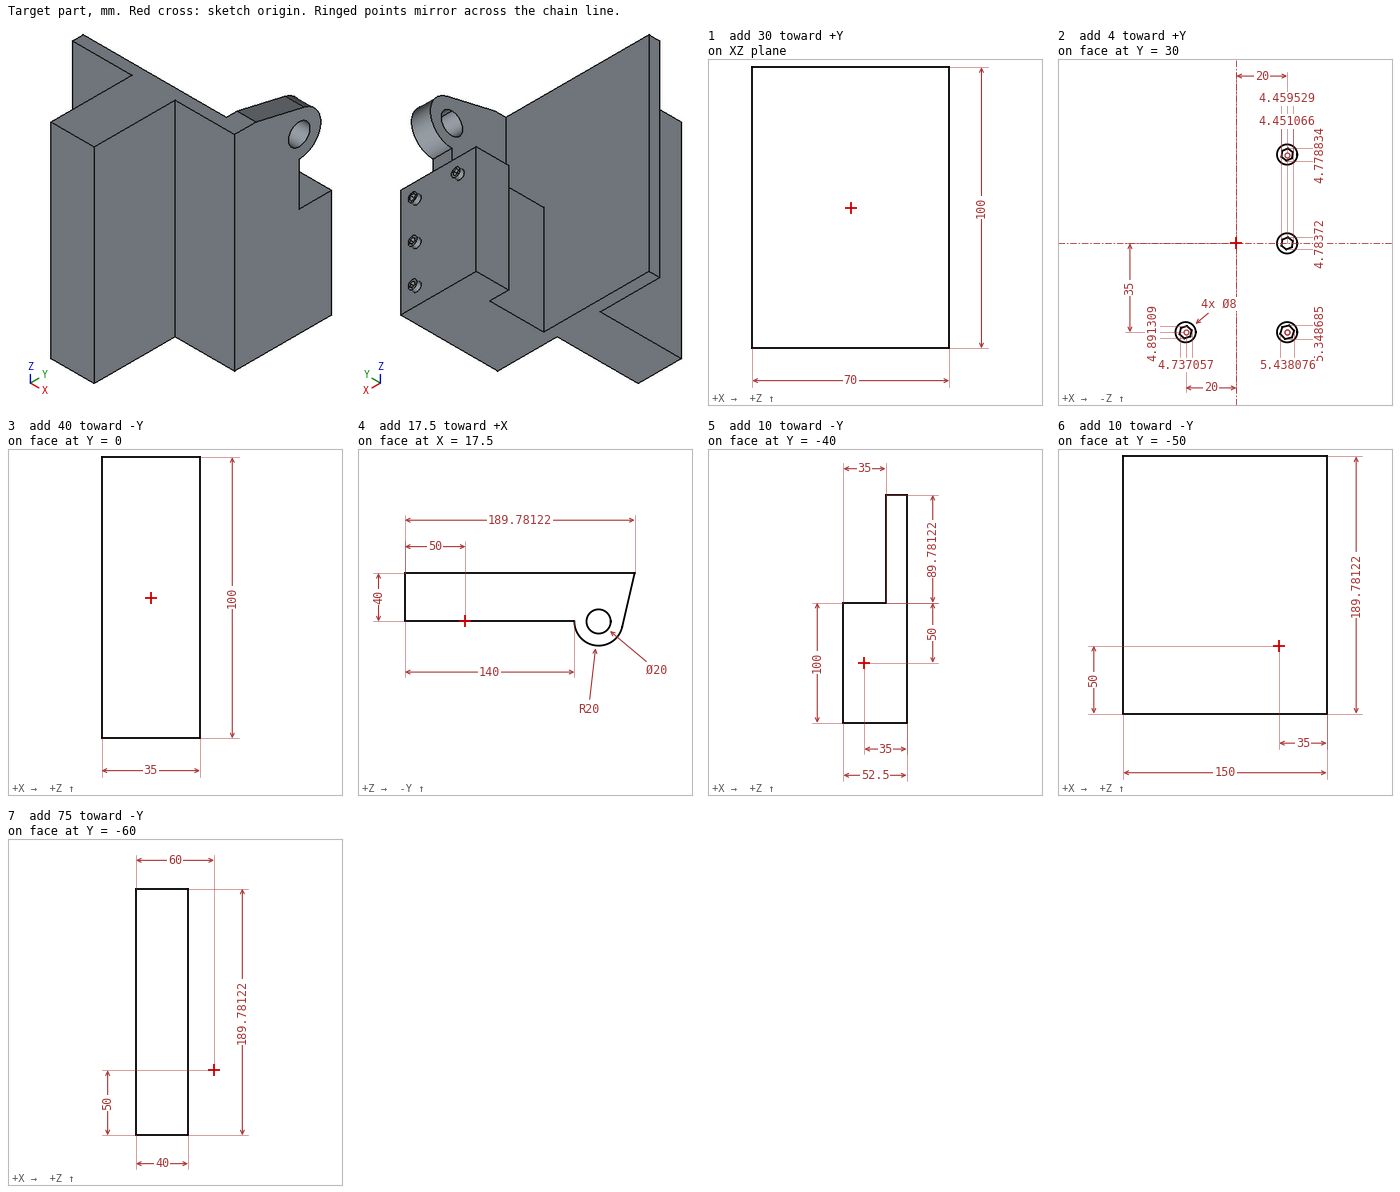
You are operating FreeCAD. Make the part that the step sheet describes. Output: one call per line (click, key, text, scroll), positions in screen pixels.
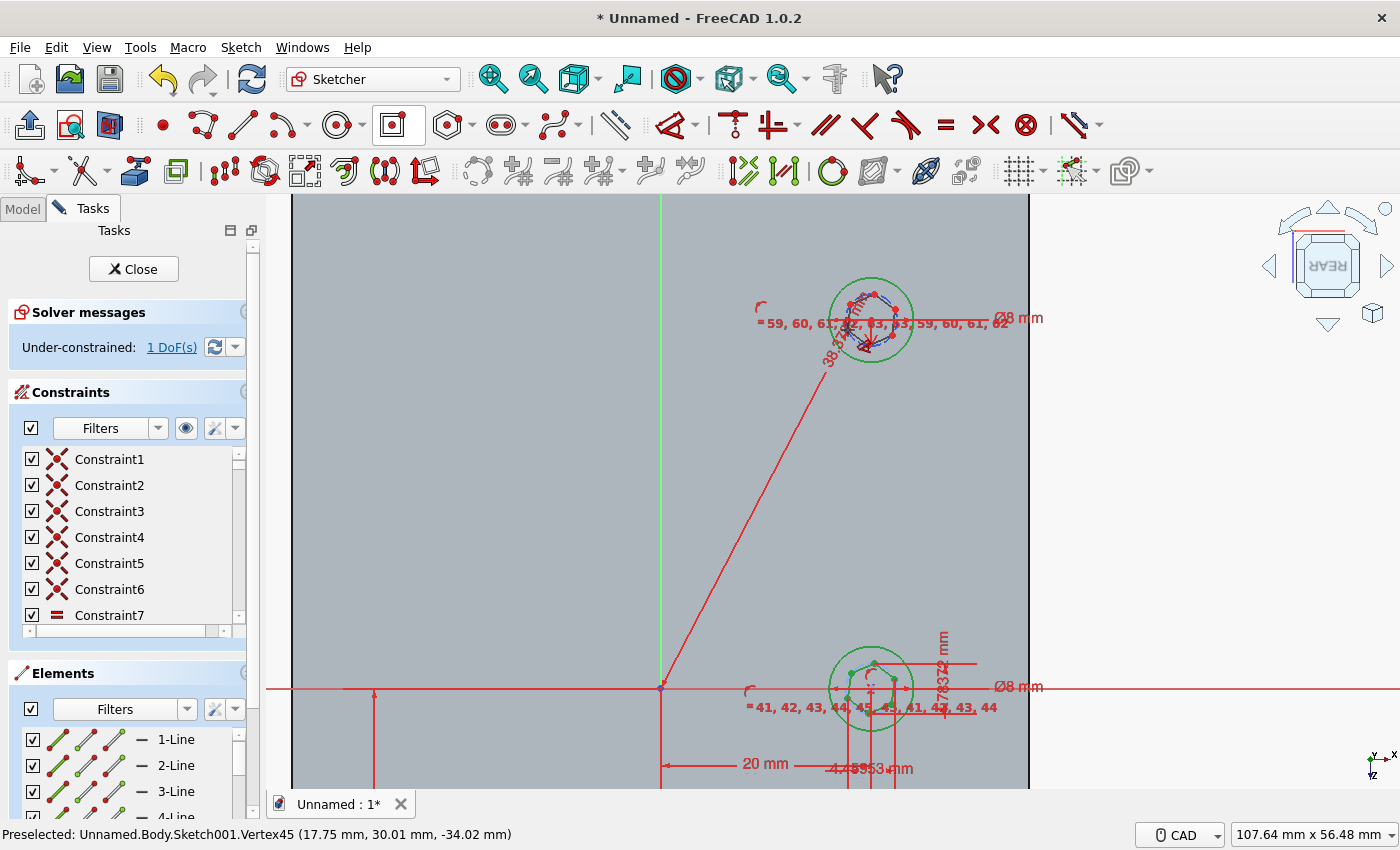
click(895, 310)
click(871, 252)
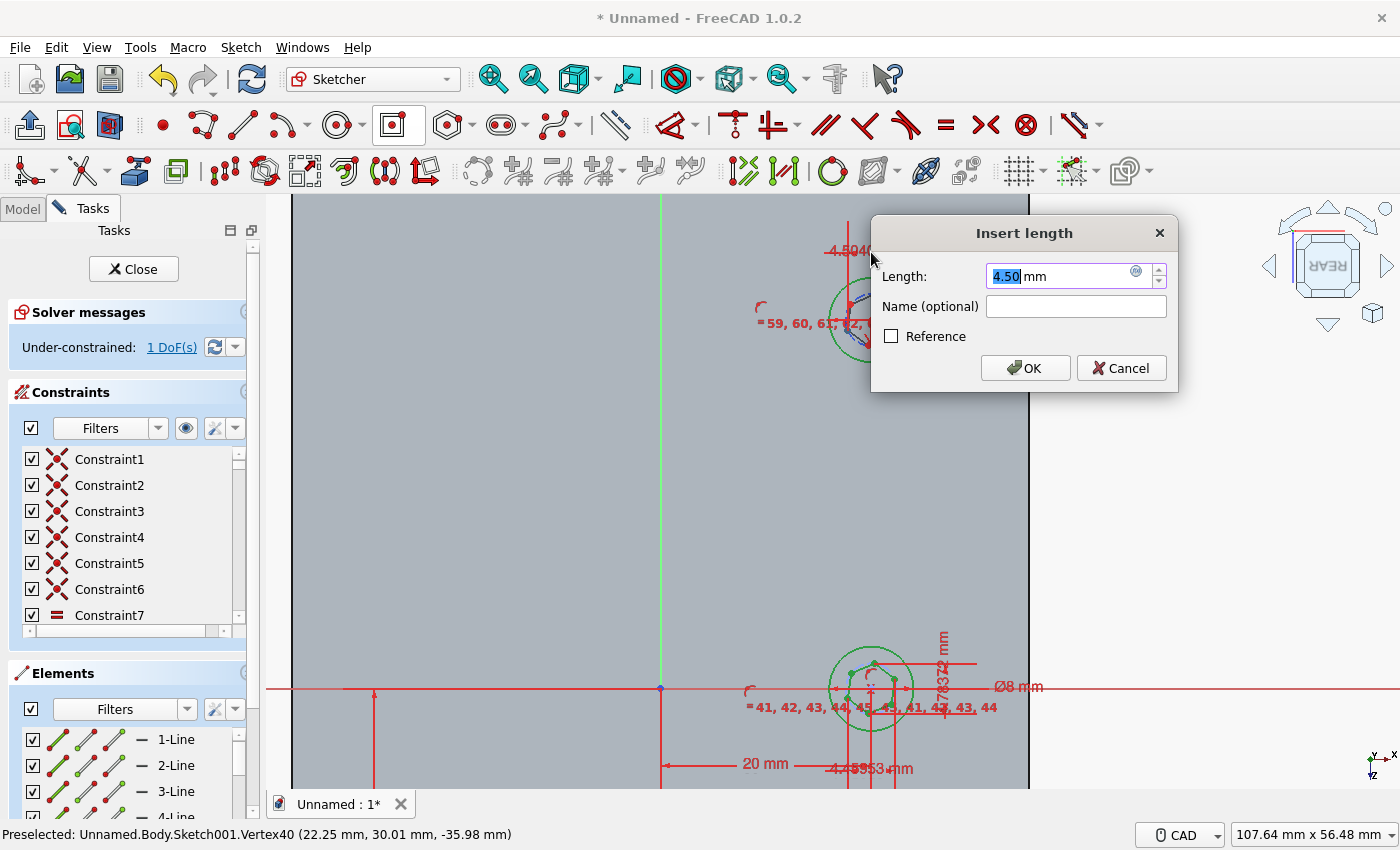
text(4.451066)
key(Return)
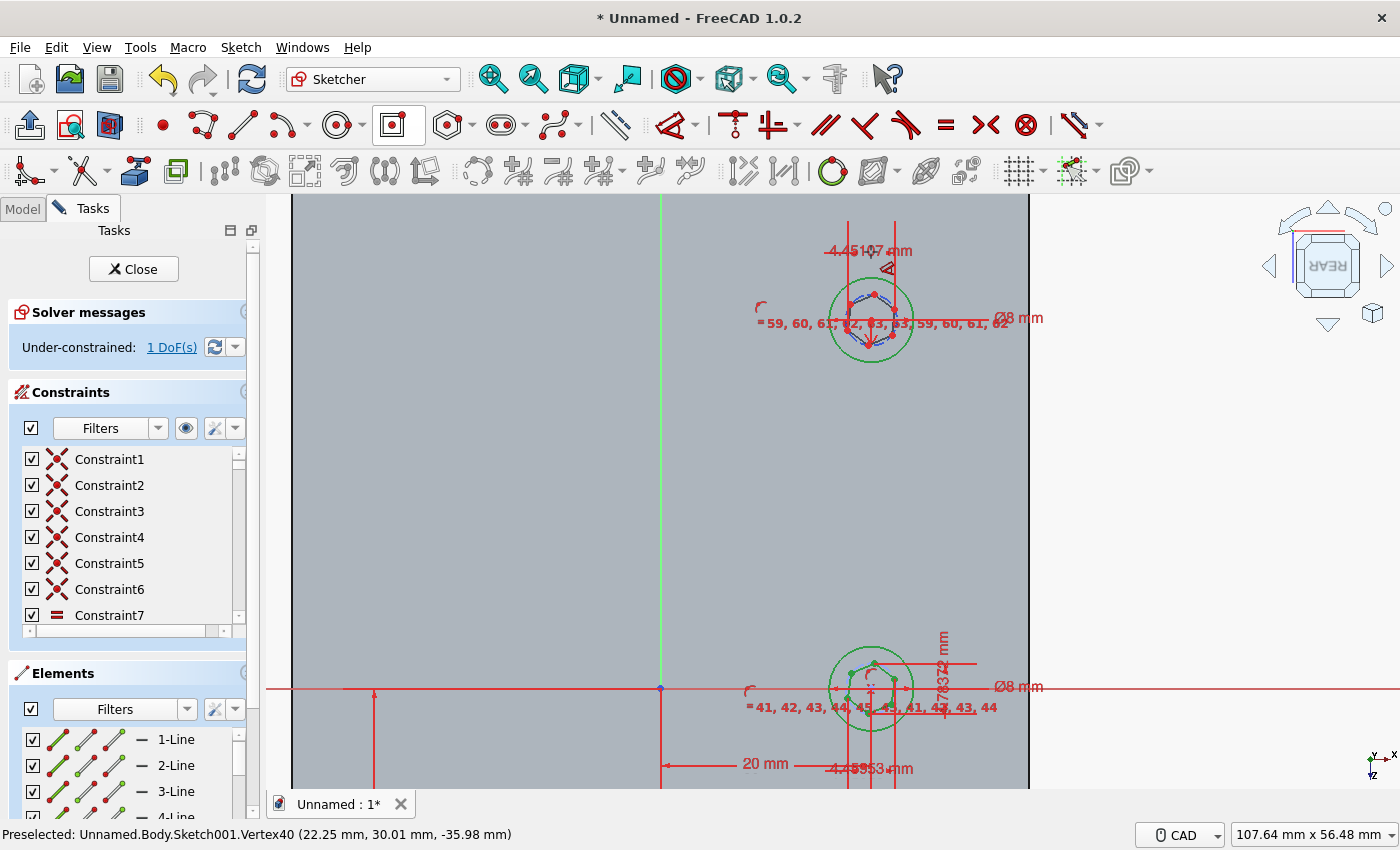
click(869, 346)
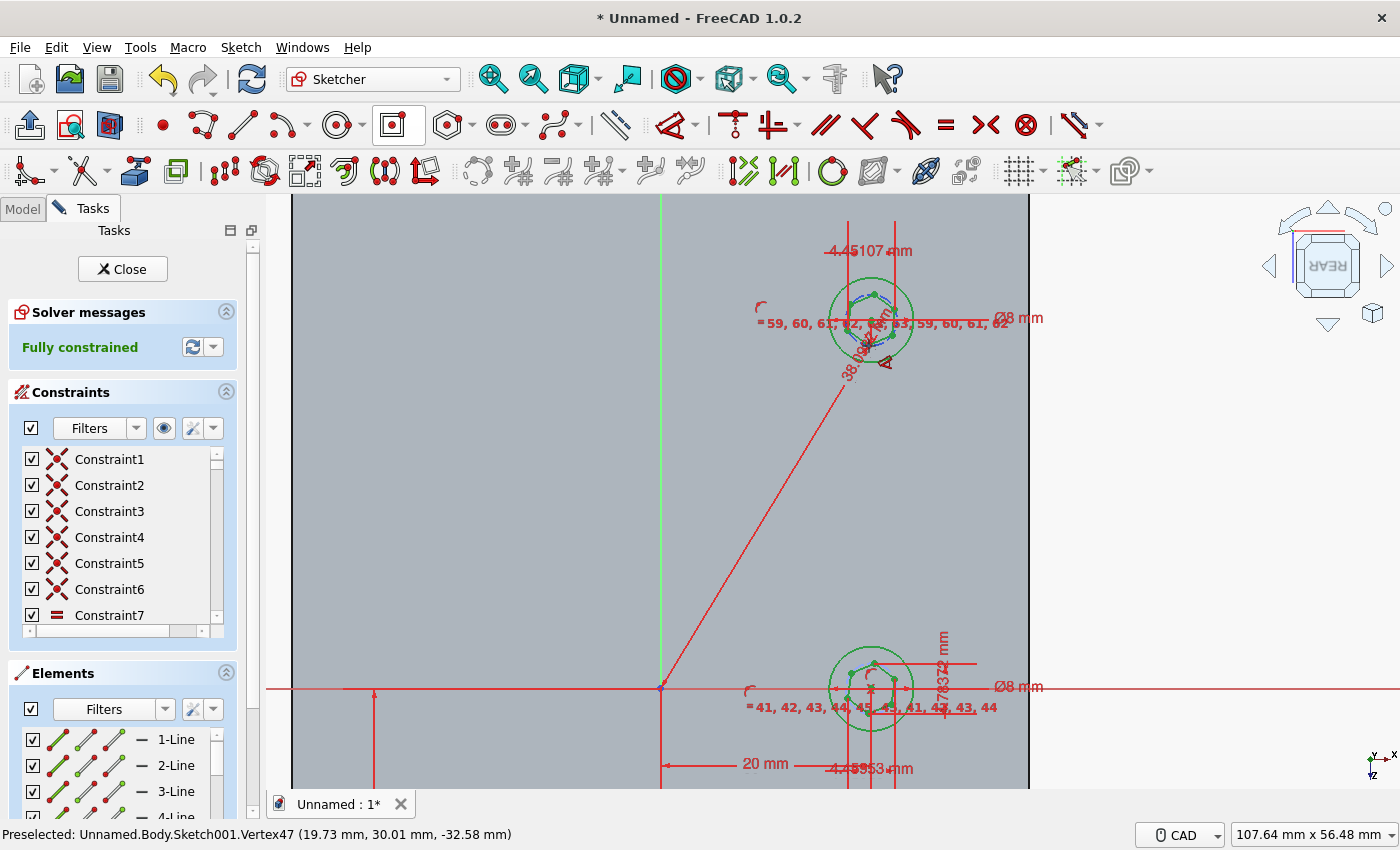
click(874, 295)
click(932, 320)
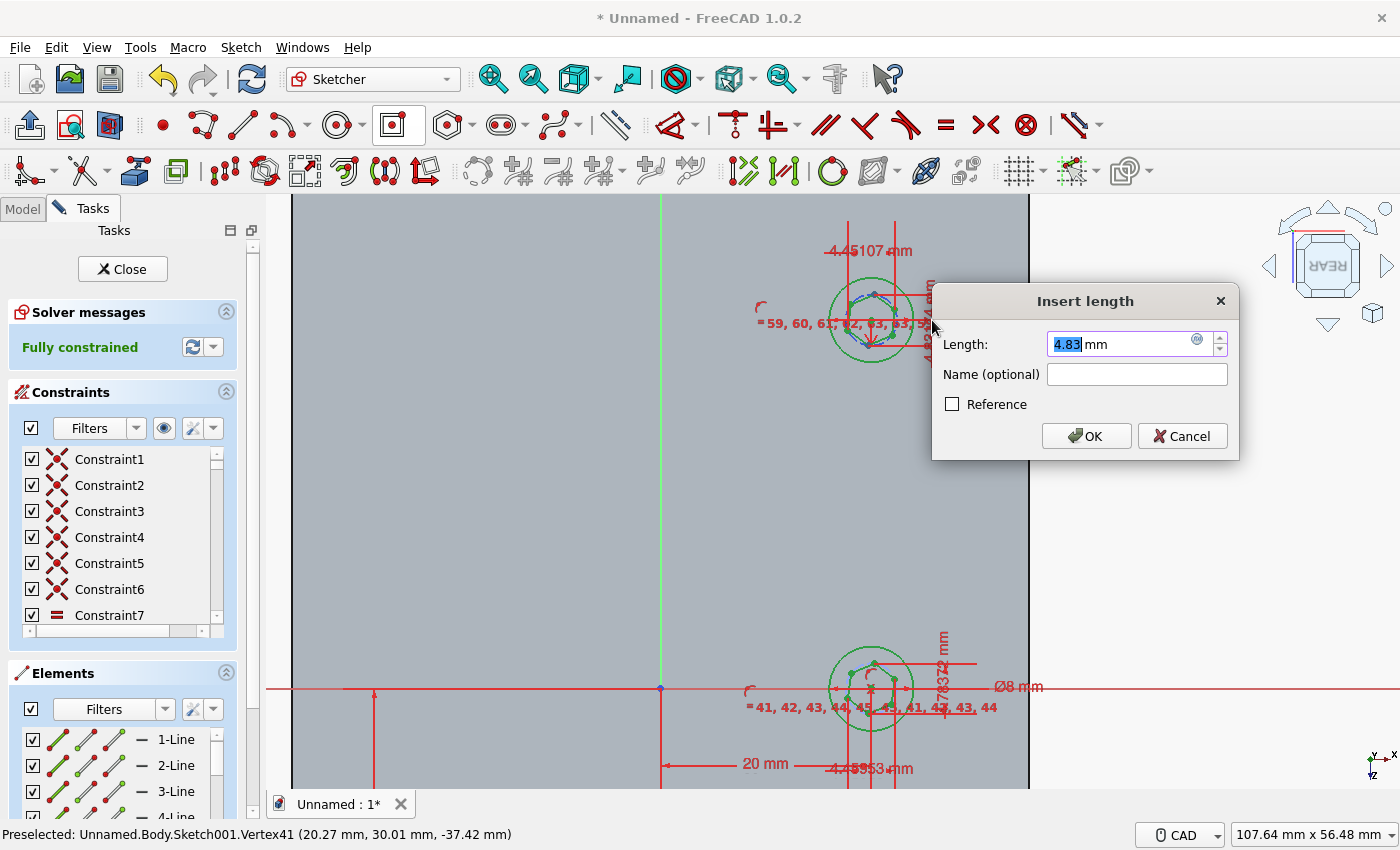
text(4.778834)
key(Return)
key(Escape)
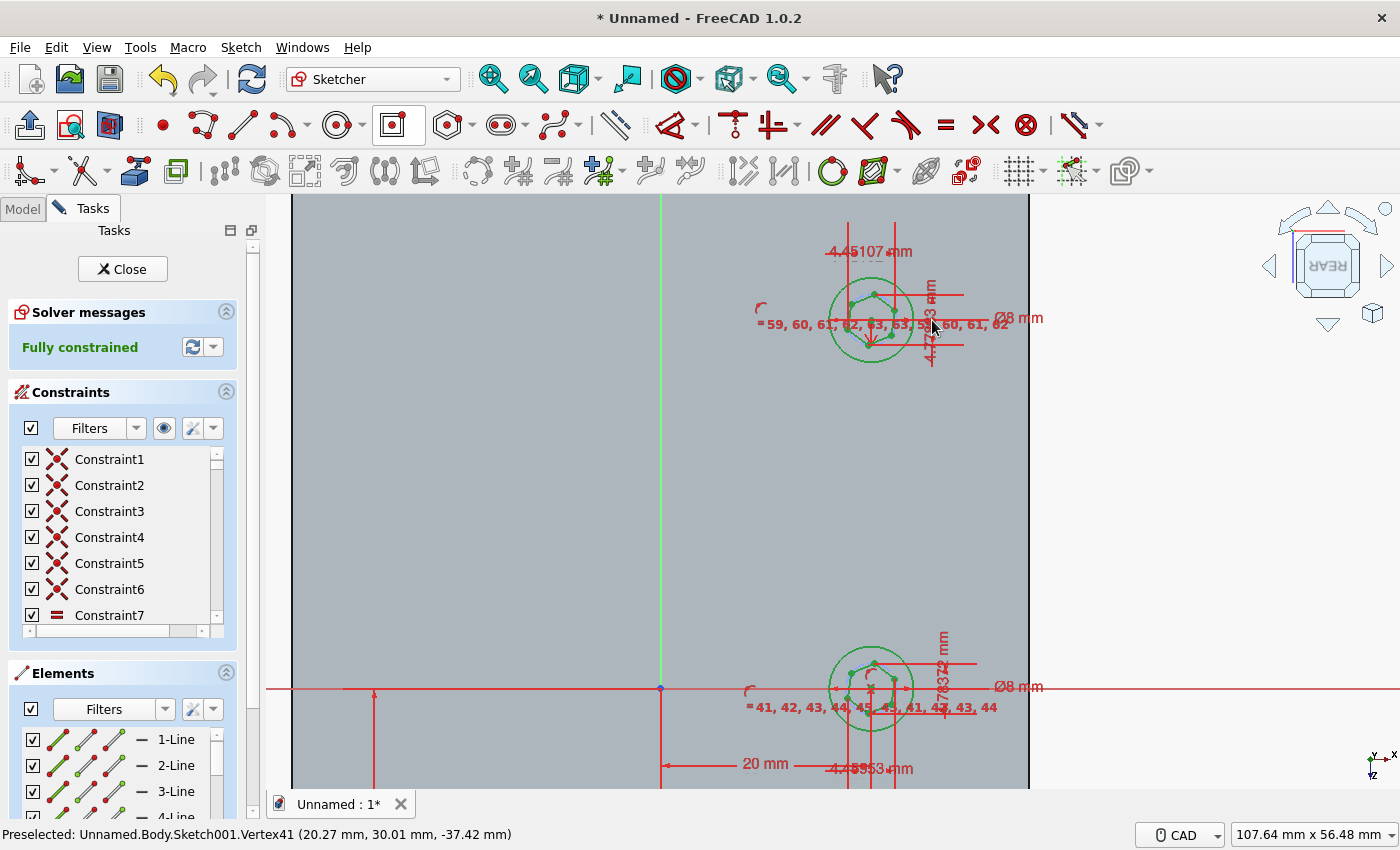
click(123, 269)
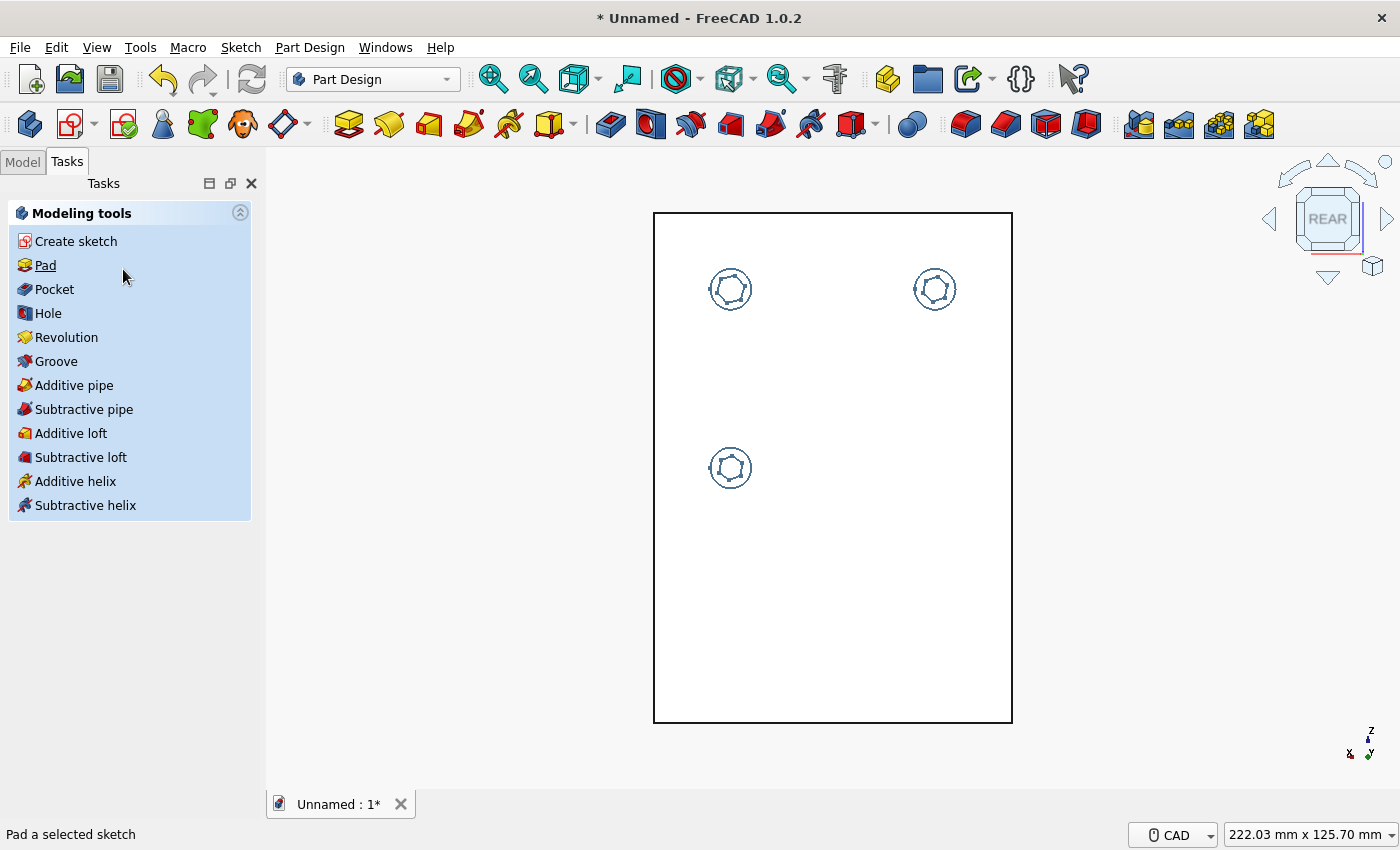
click(350, 124)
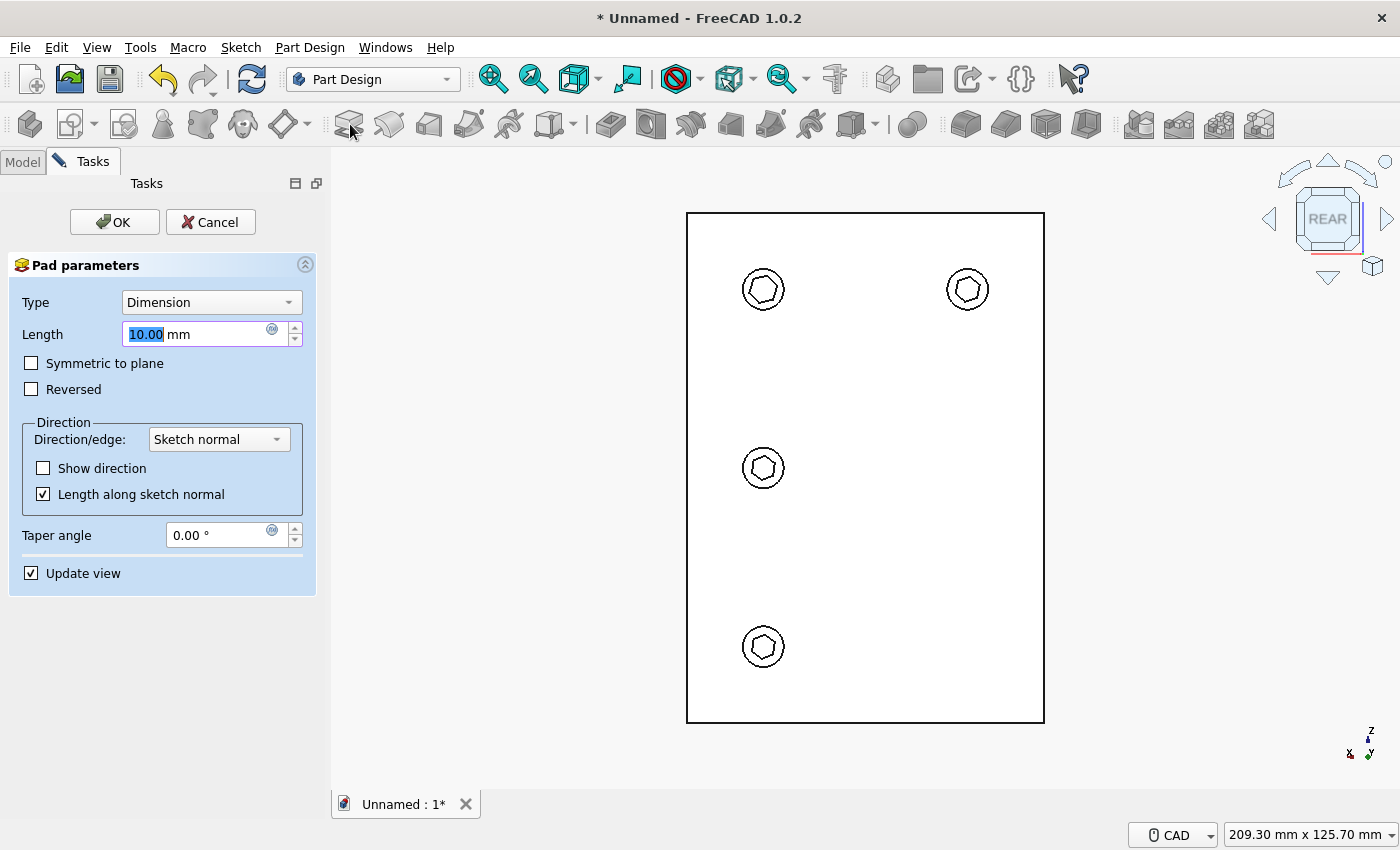
text(4)
key(Tab)